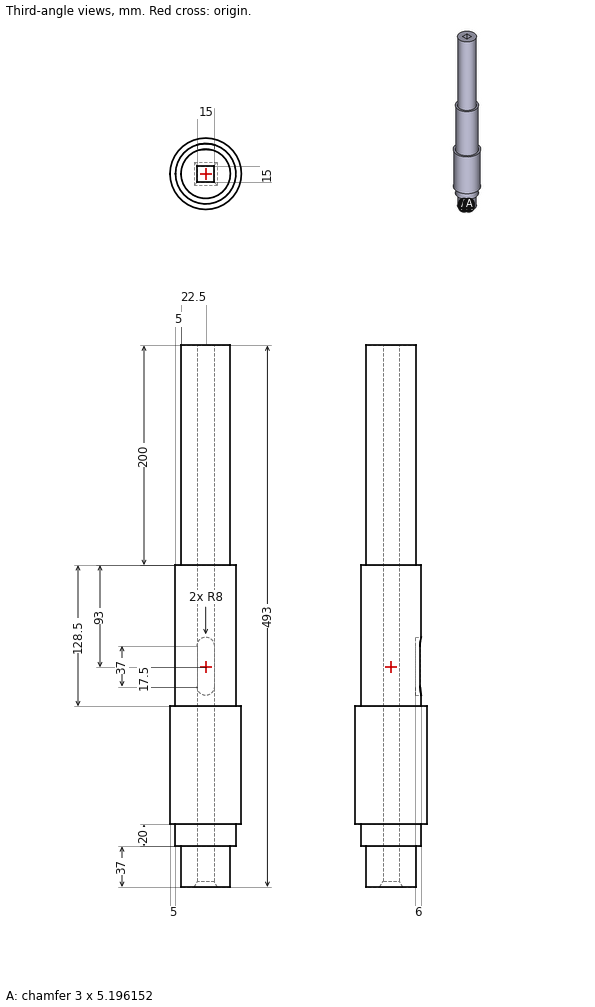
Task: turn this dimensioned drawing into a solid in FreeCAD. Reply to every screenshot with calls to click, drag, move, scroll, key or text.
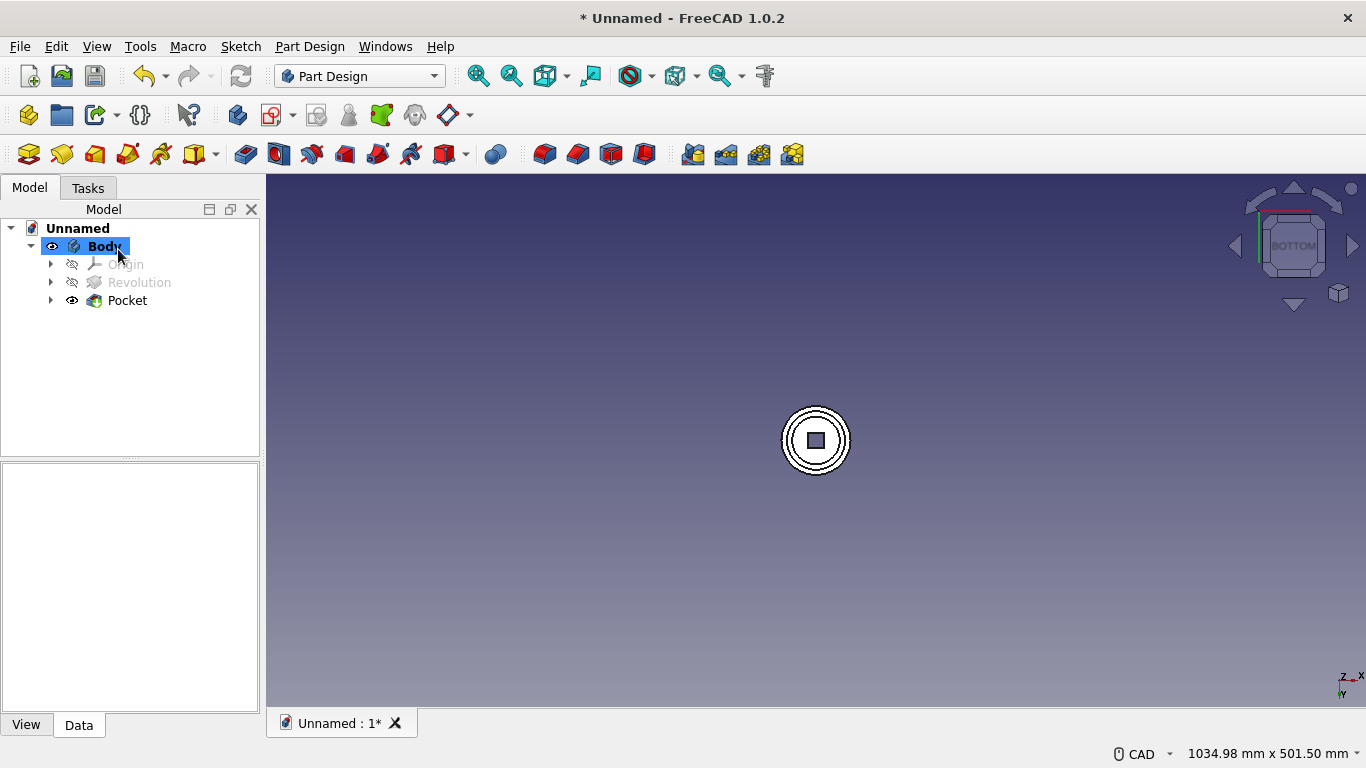
click(479, 76)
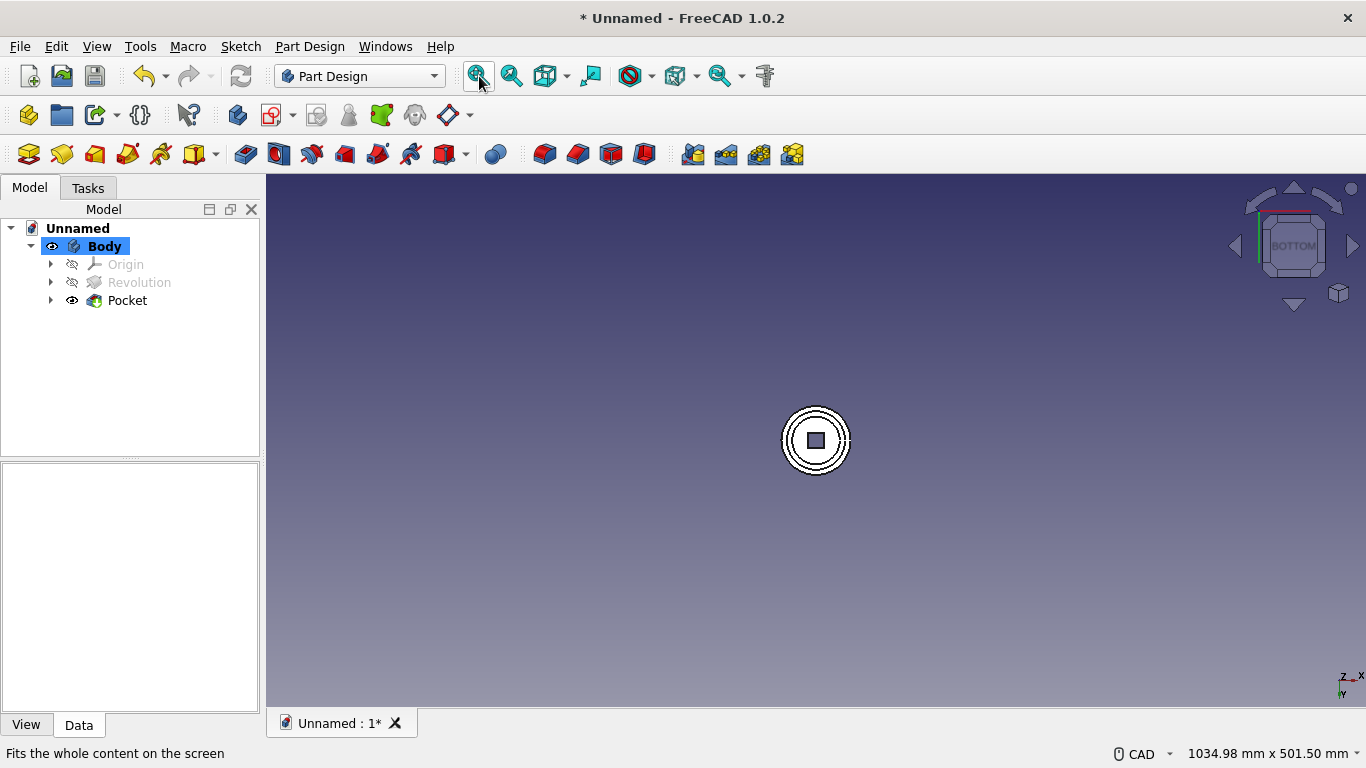
click(824, 439)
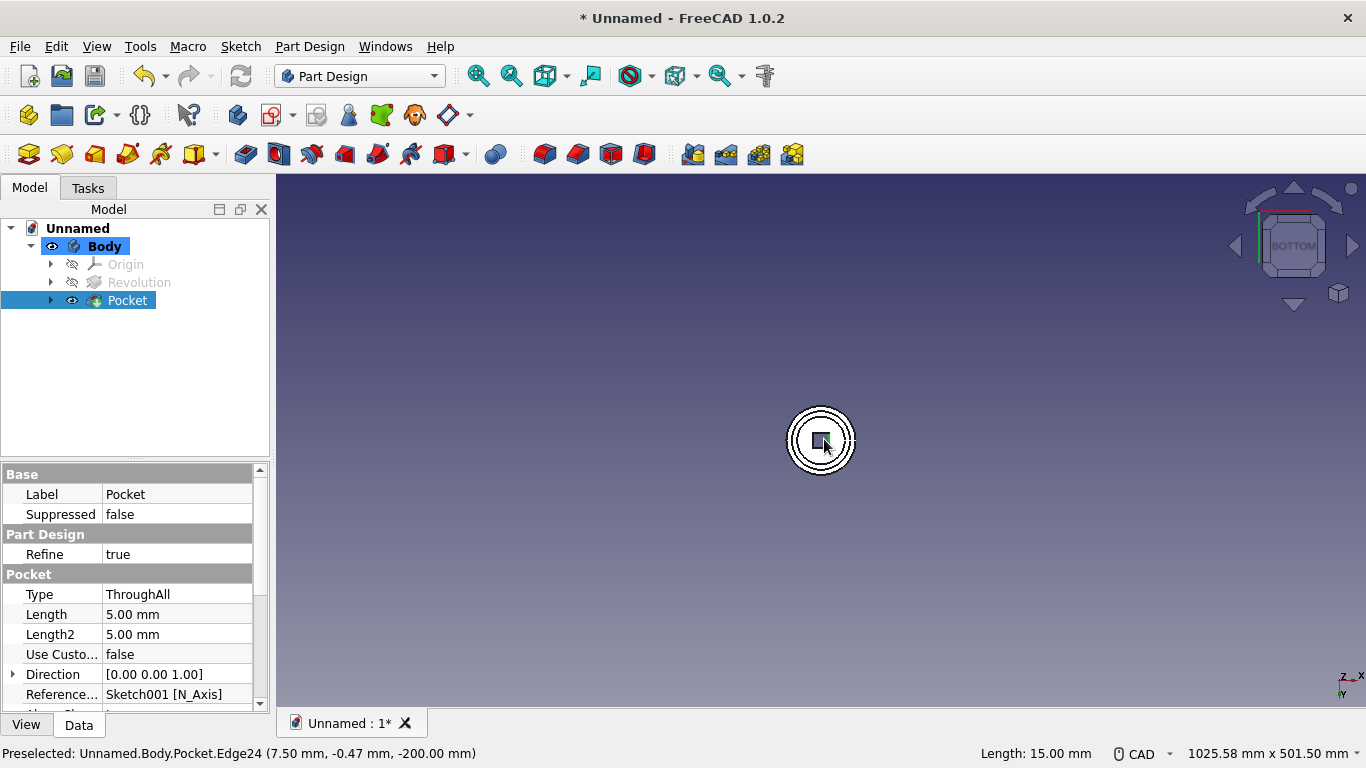
click(813, 439, ctrl)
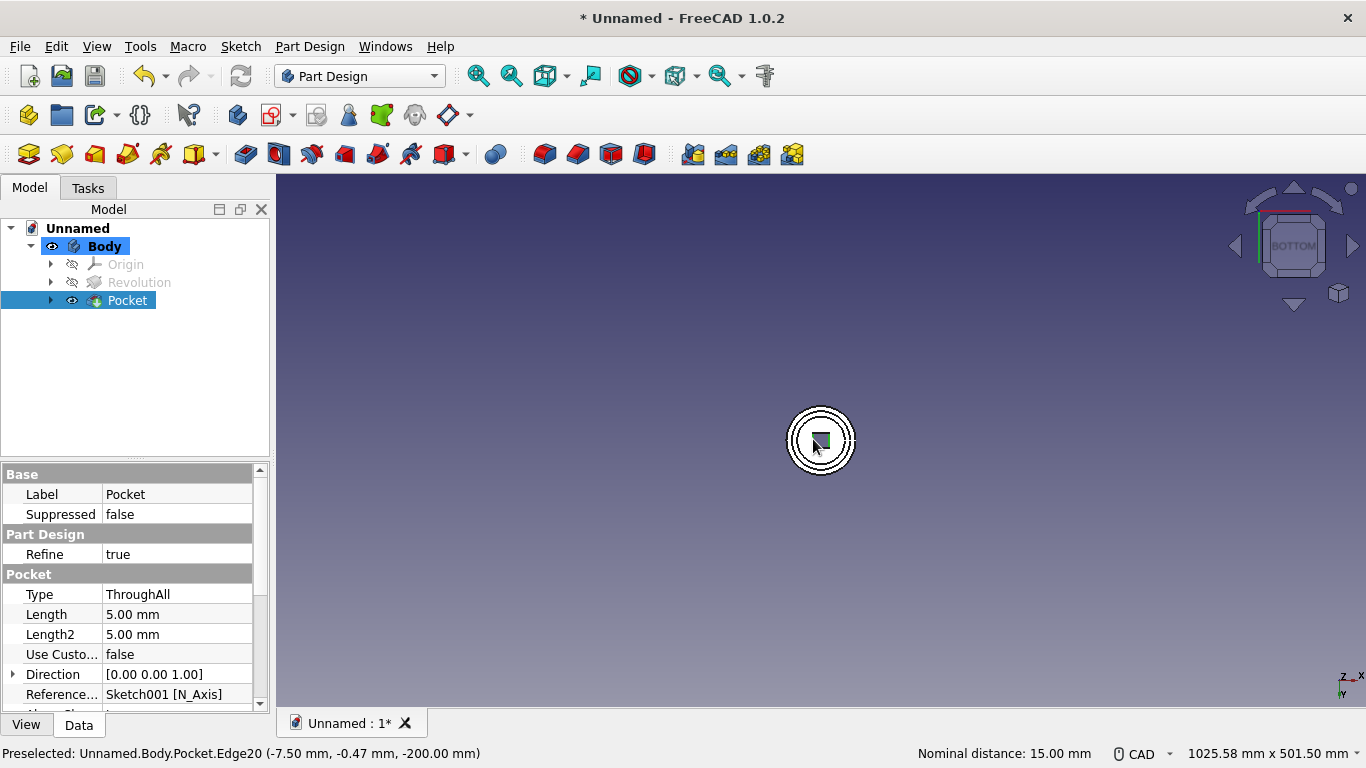
click(821, 447, ctrl)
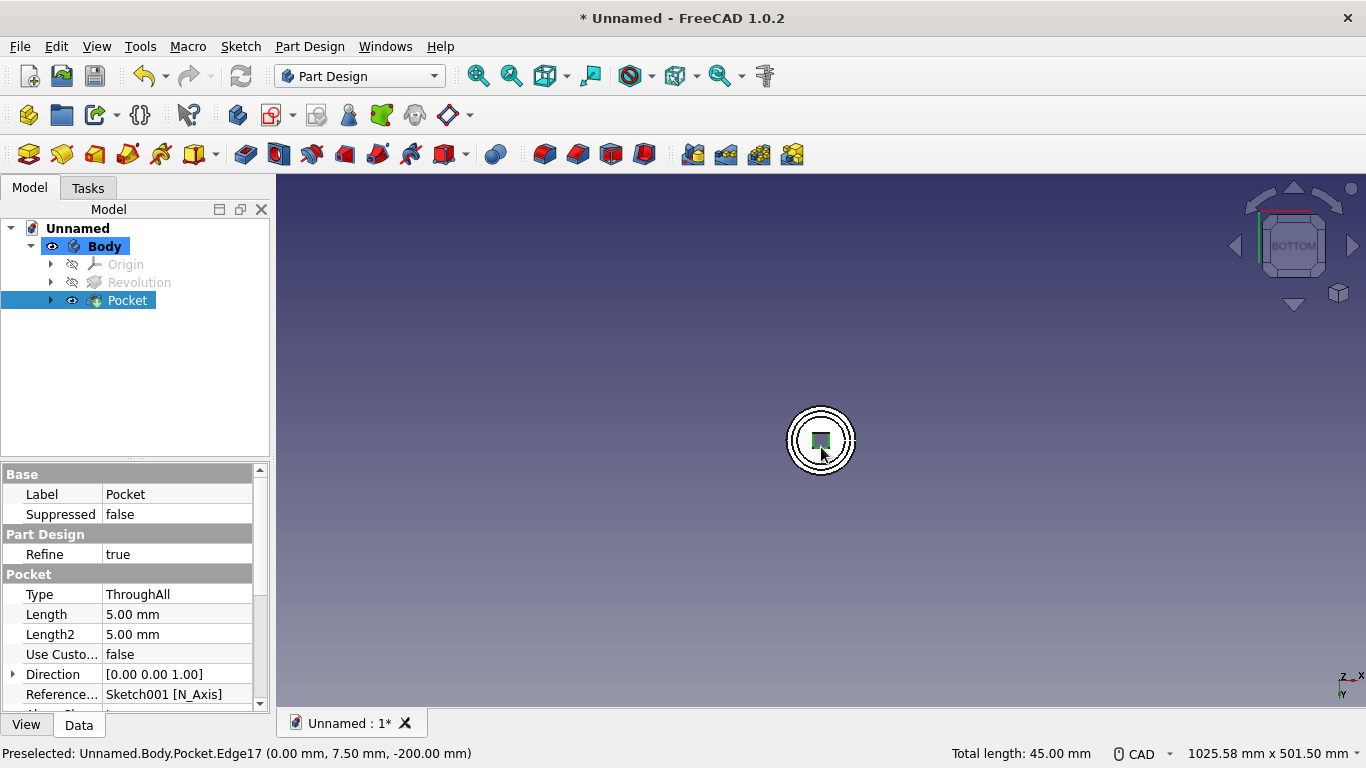
scroll(821, 432, up, 5)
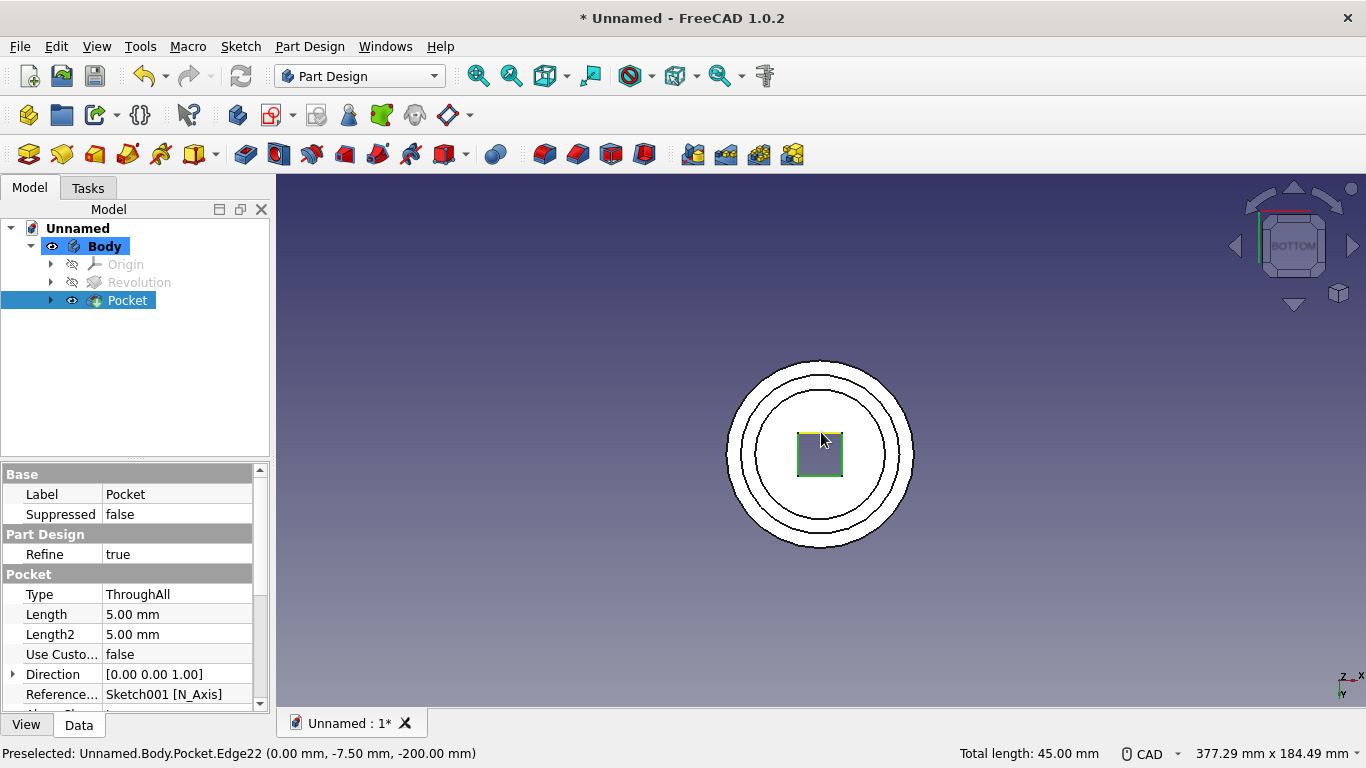
click(479, 76)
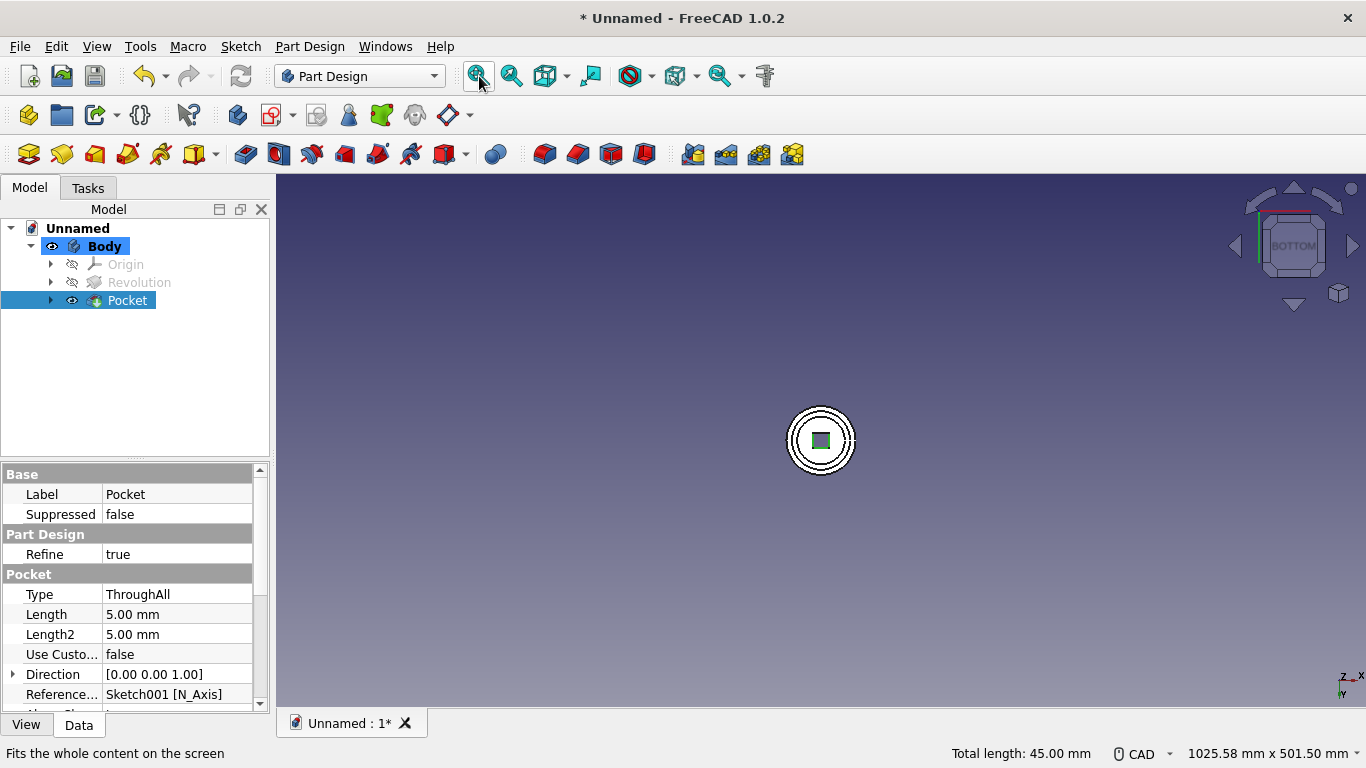
key(0)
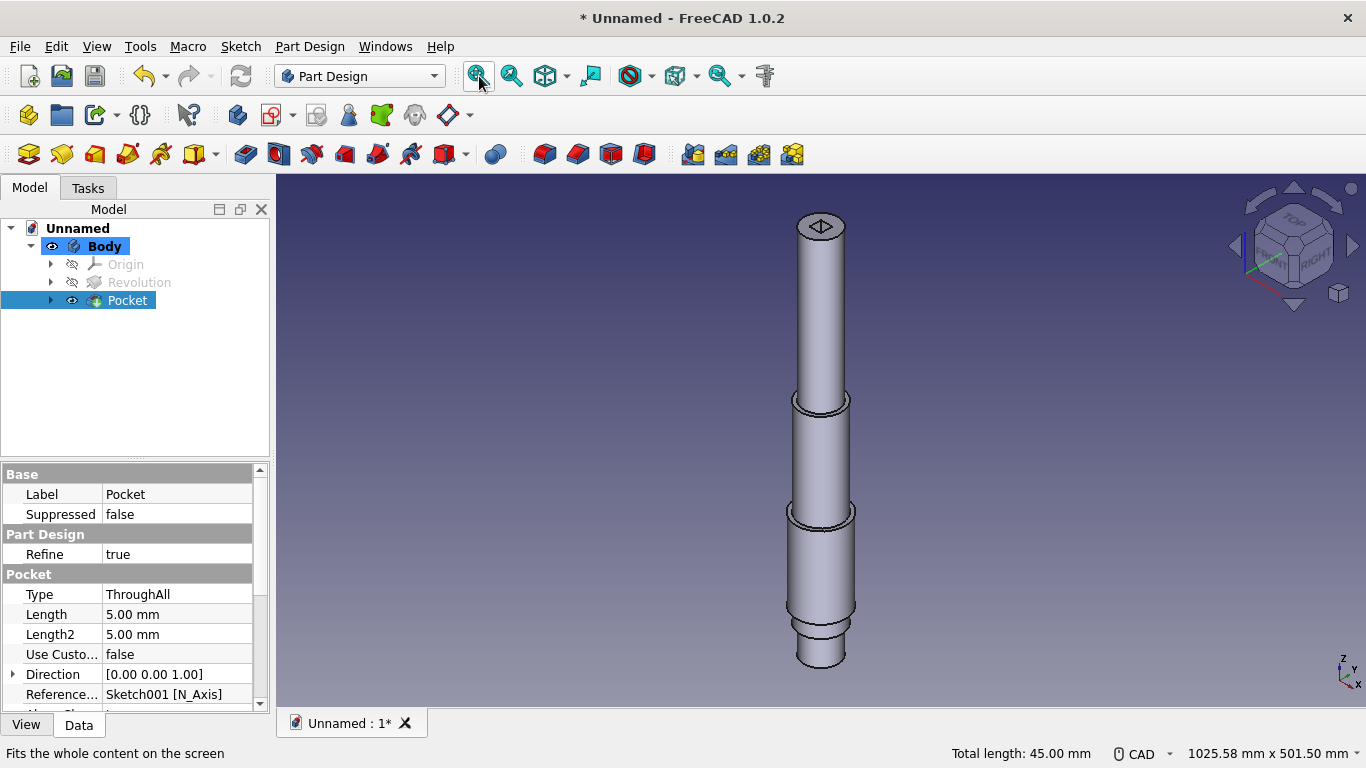
scroll(815, 657, up, 5)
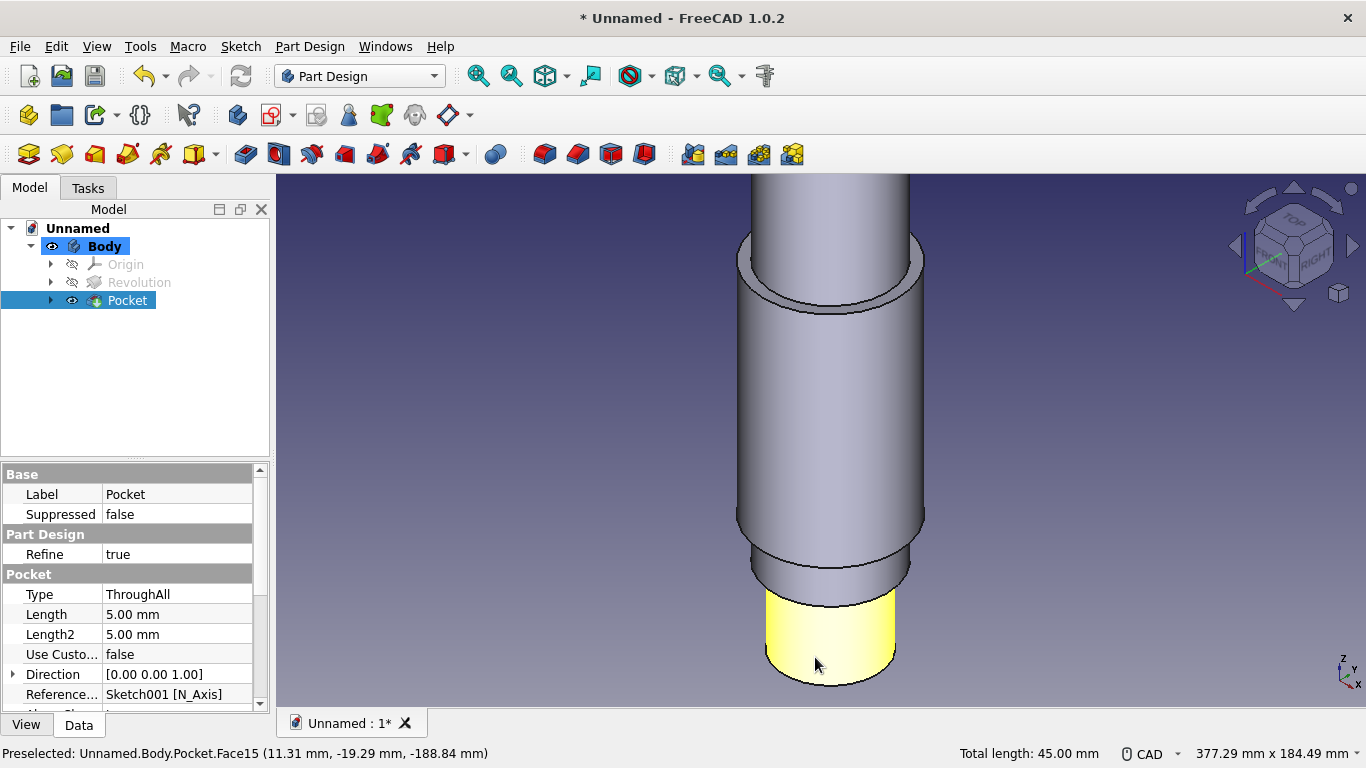
click(479, 76)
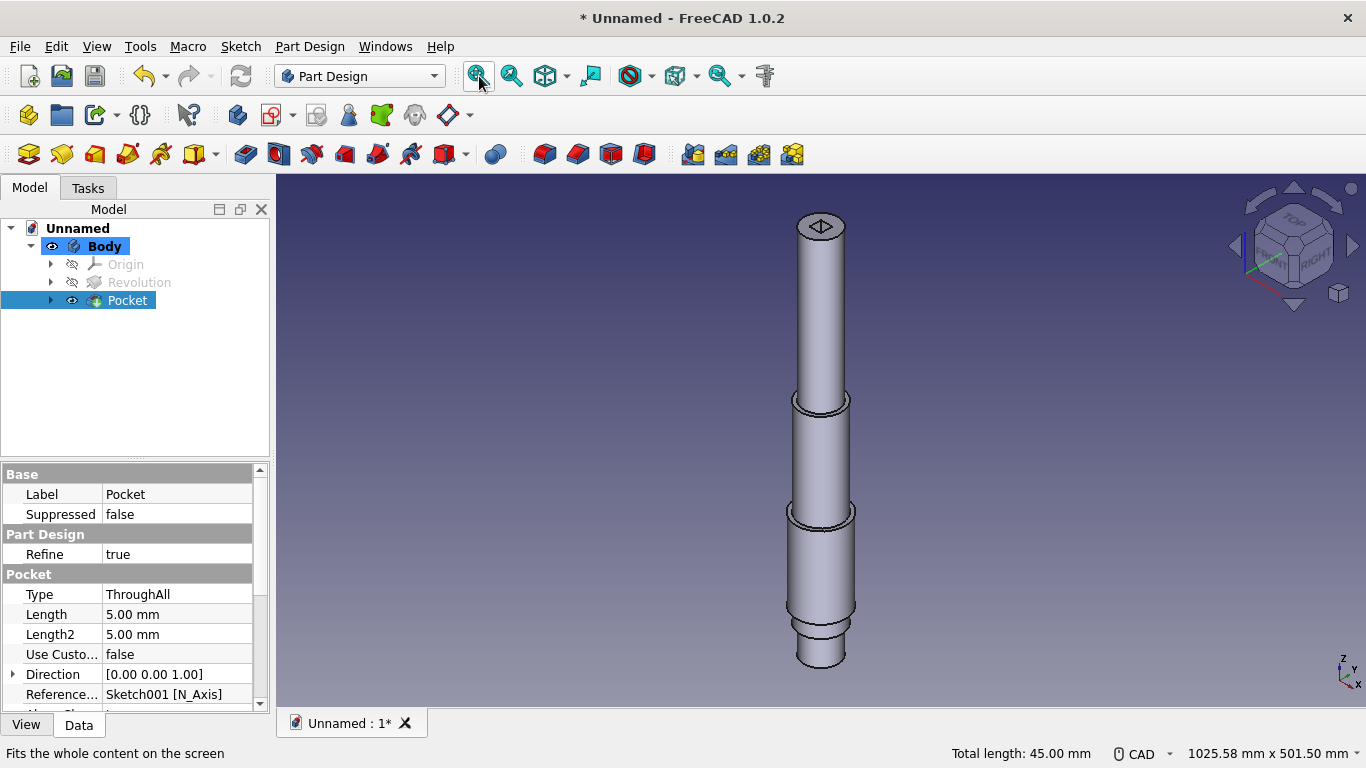
key(2)